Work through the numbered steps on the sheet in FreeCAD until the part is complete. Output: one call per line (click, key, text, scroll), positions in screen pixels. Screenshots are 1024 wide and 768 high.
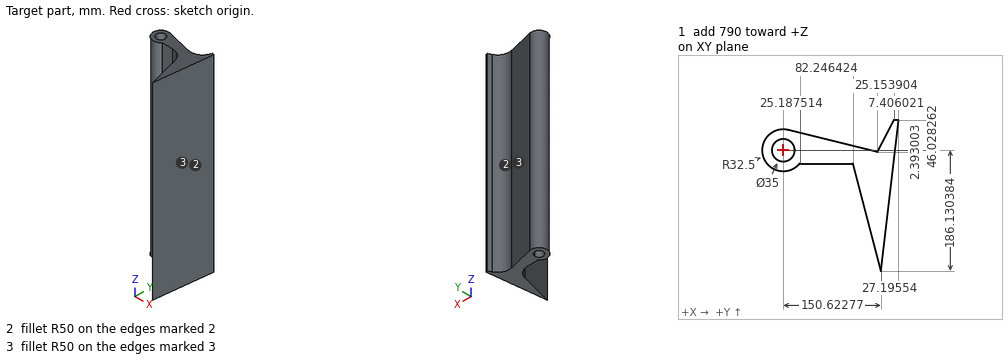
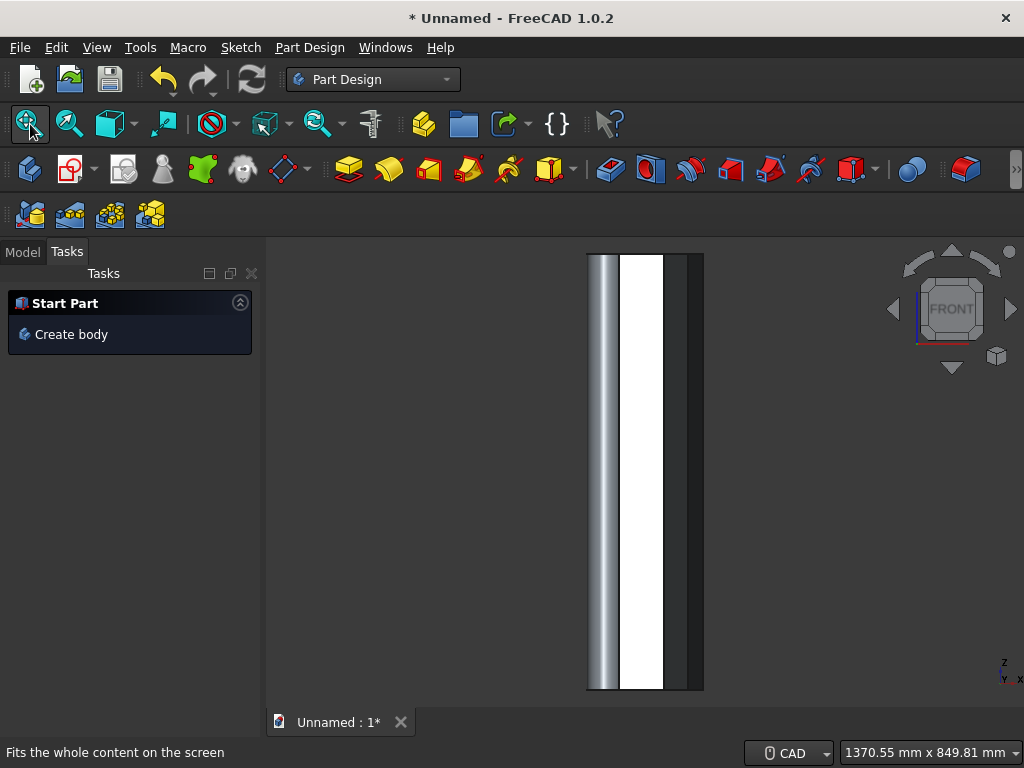
key(3)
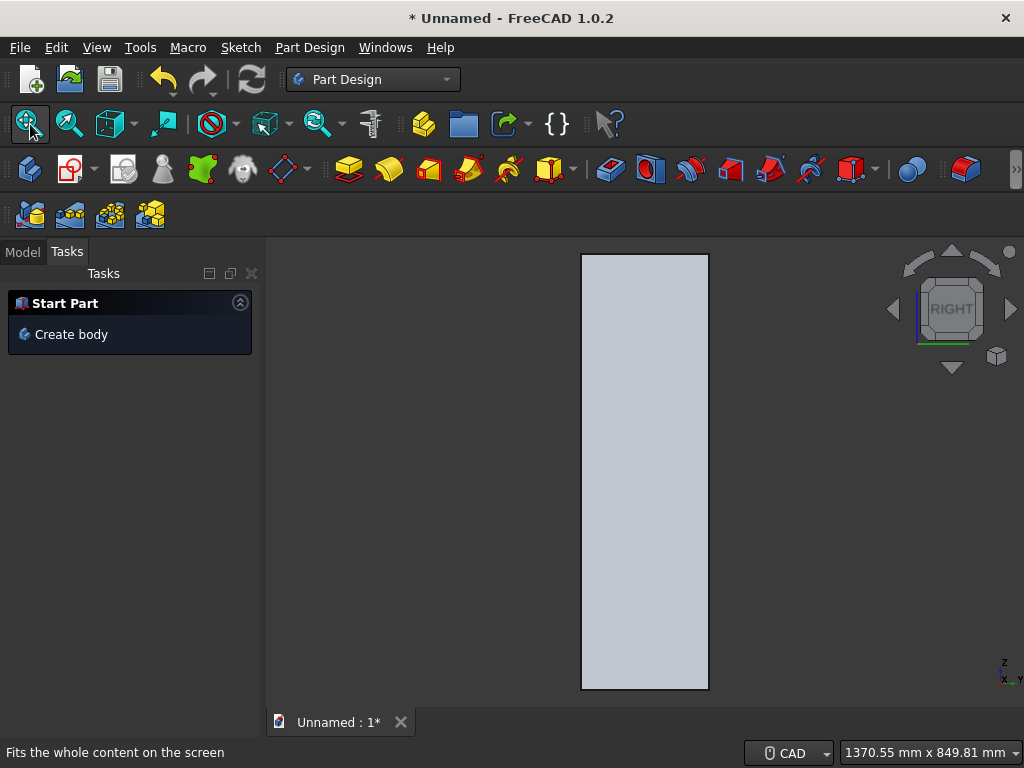
key(5)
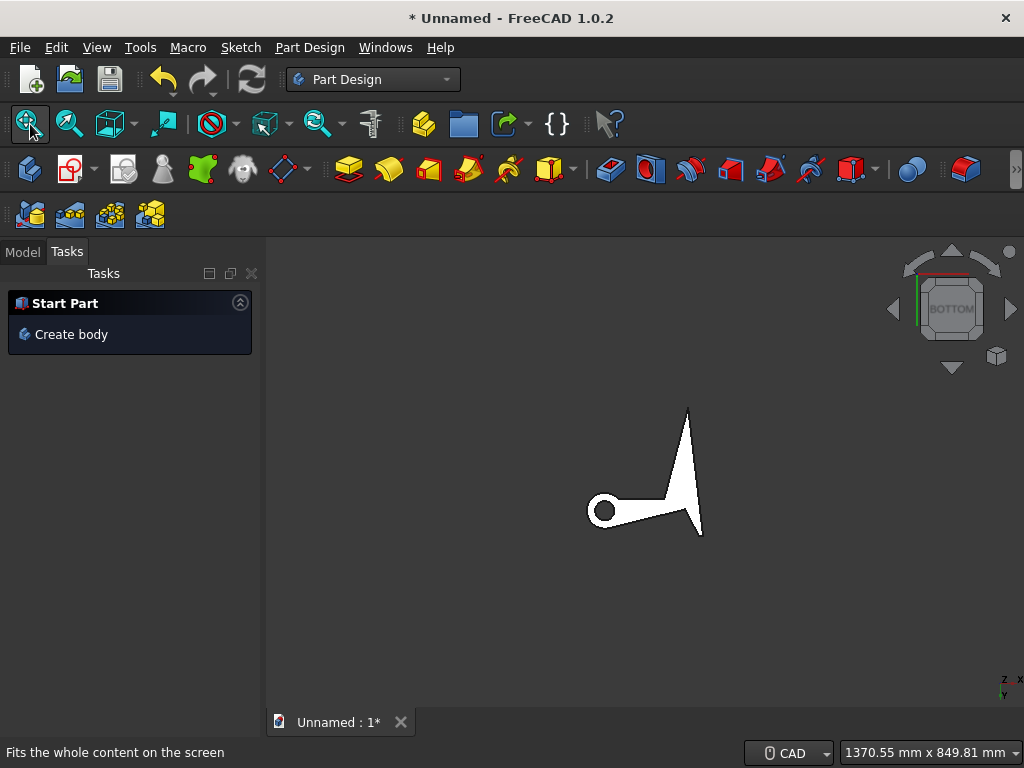
key(v)
key(f)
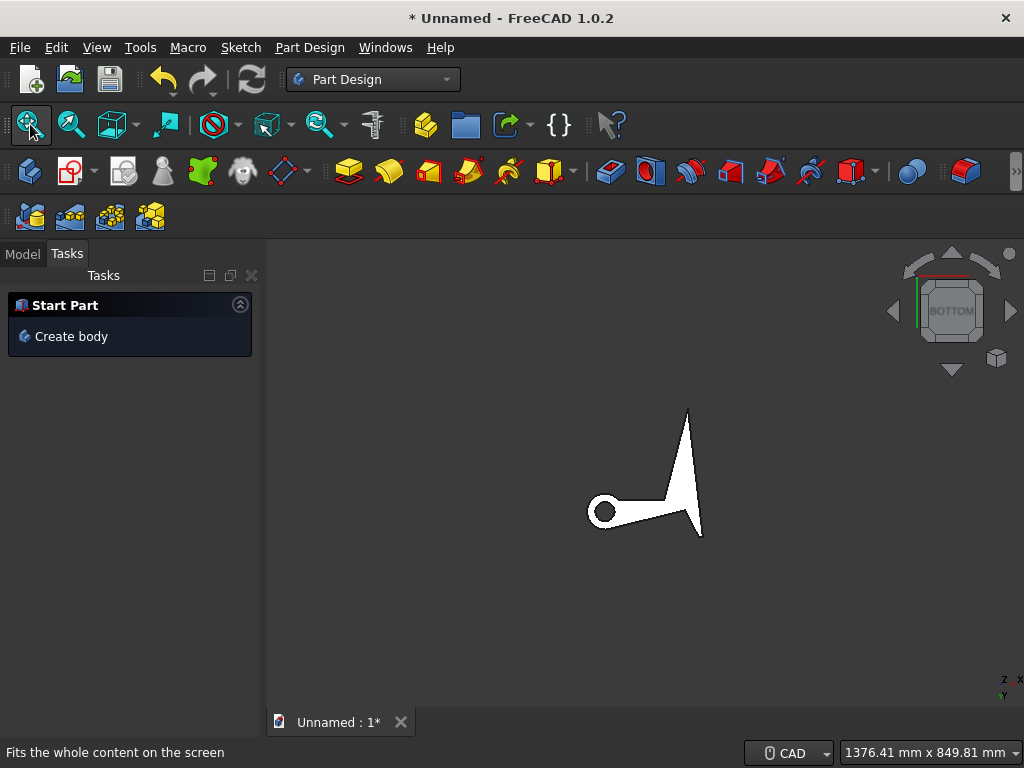
key(4)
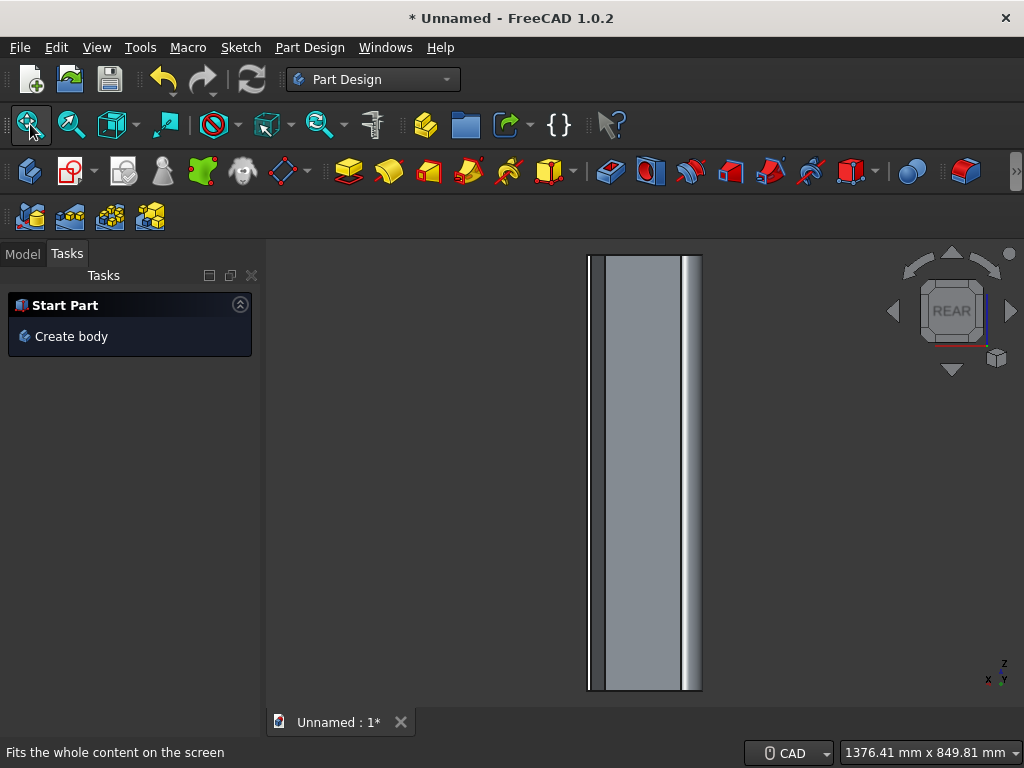
key(6)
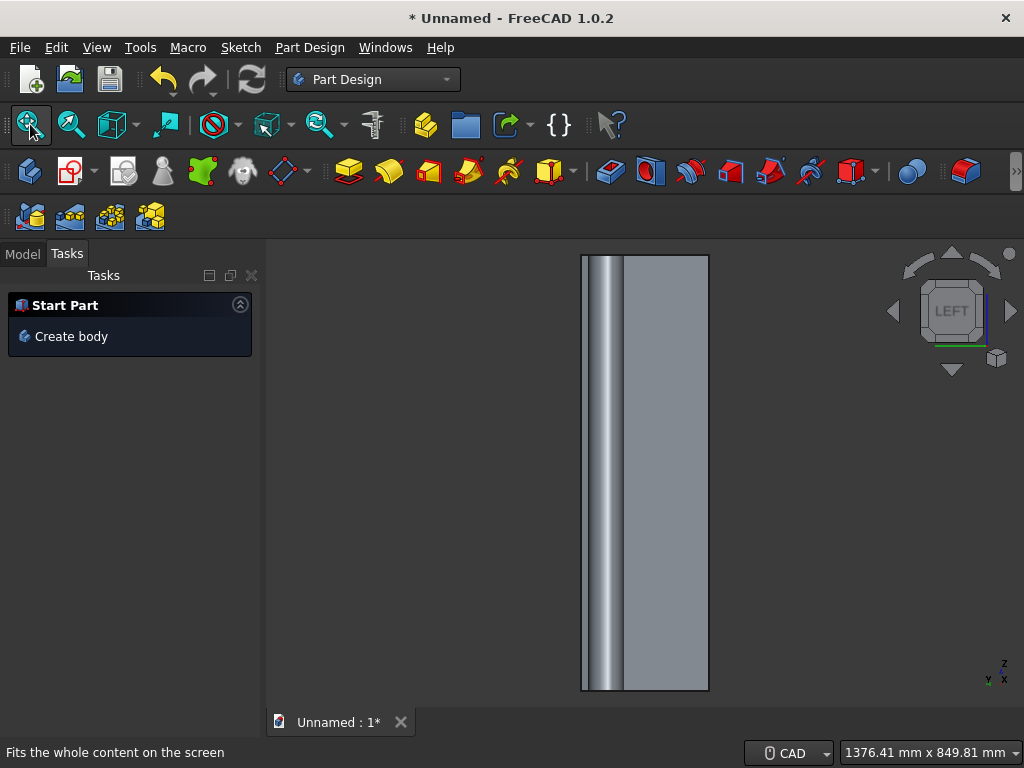
key(v)
key(3)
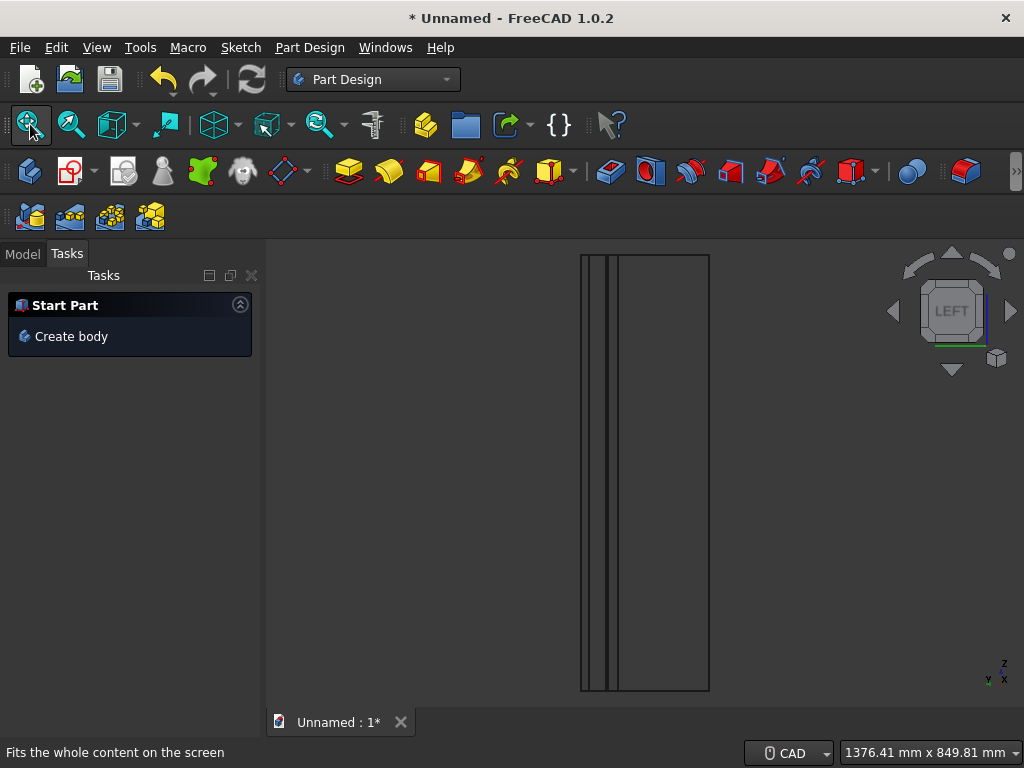
key(0)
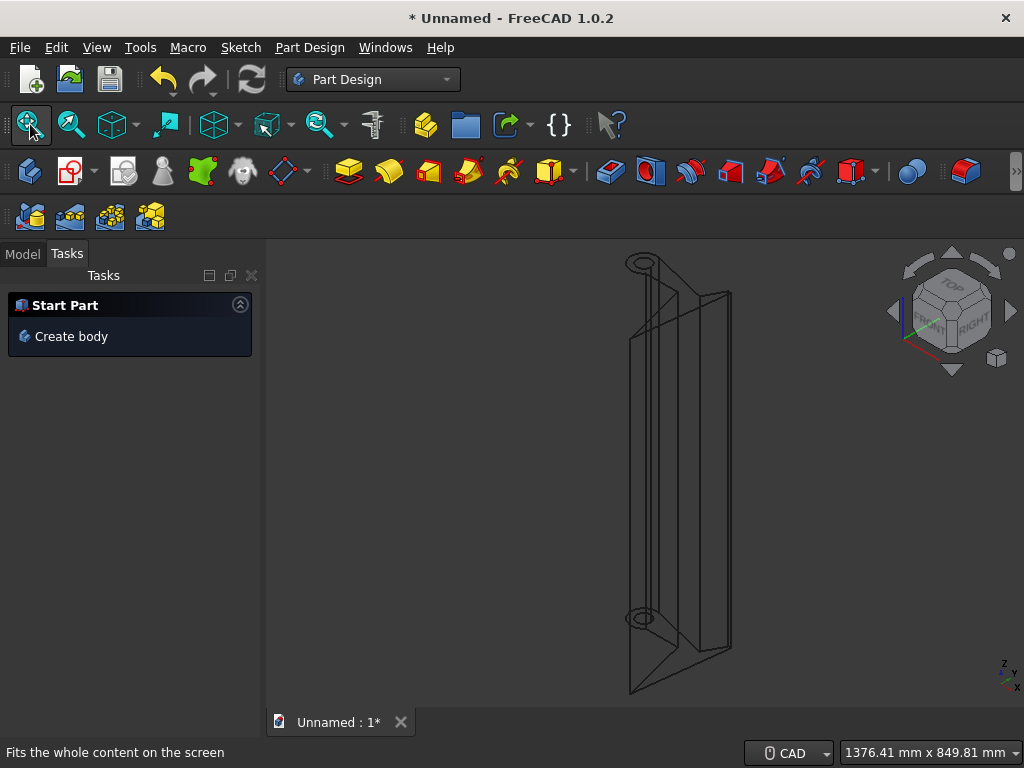
click(700, 473)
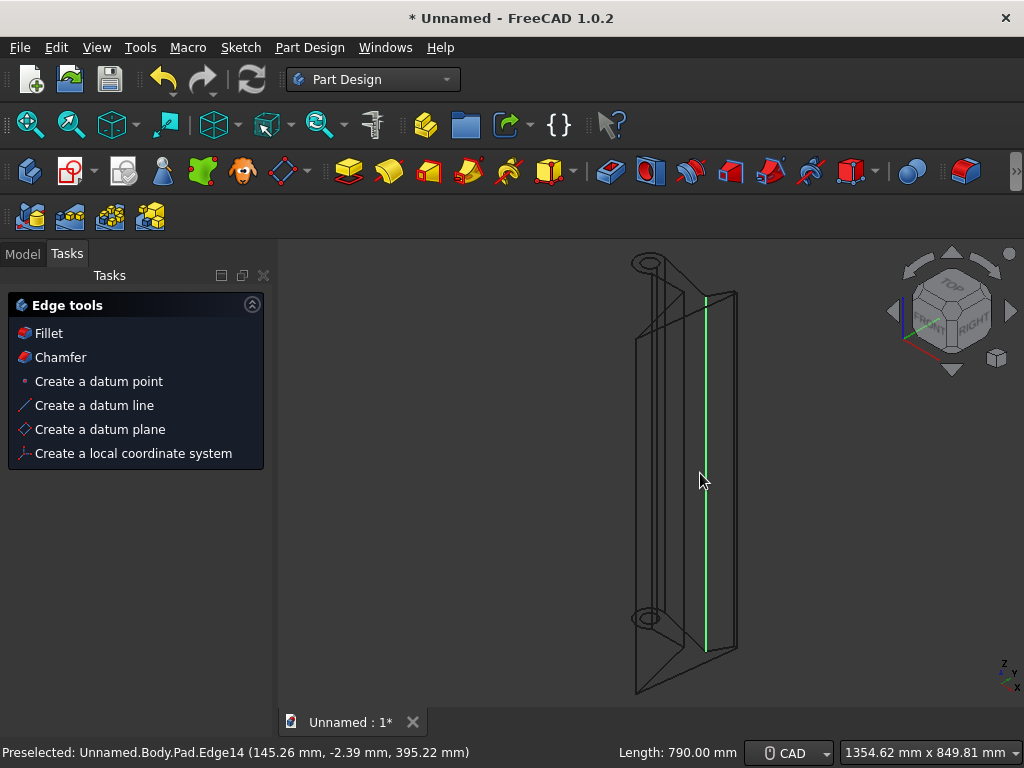
key(v)
key(1)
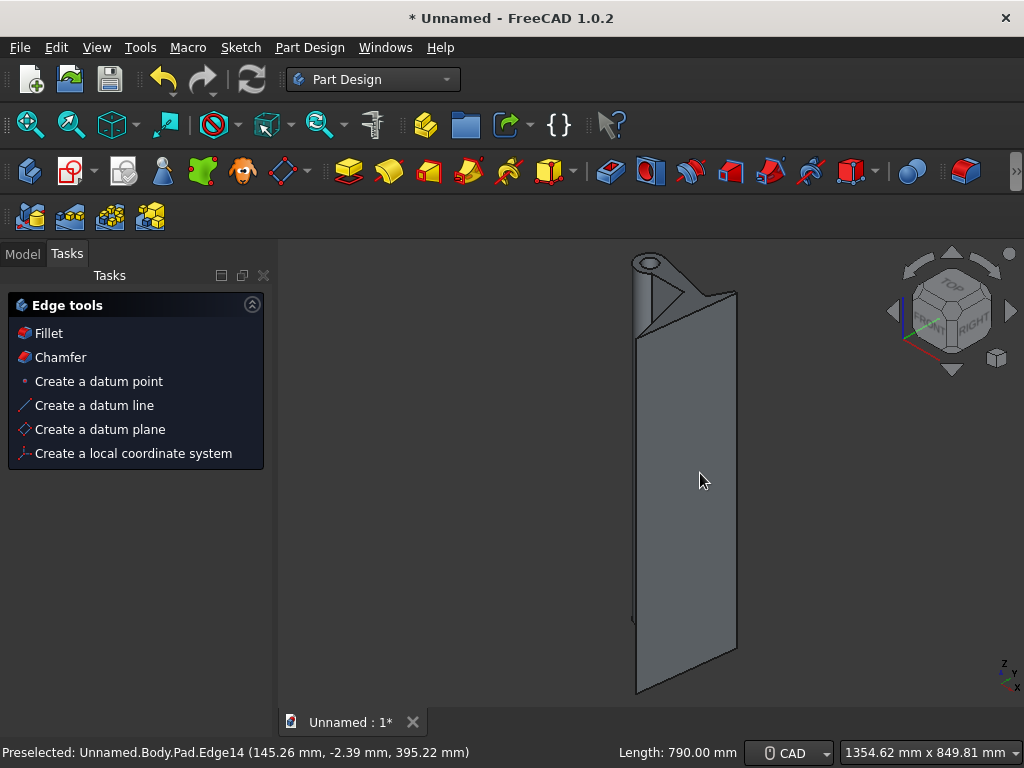
click(966, 172)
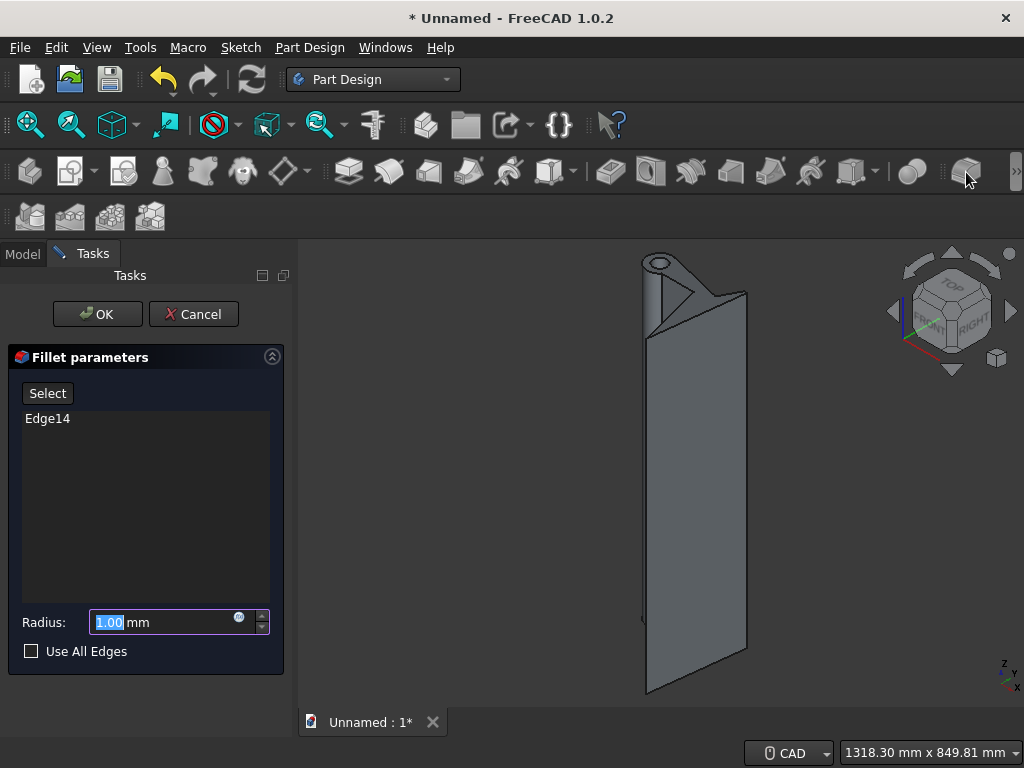
text(50)
key(Tab)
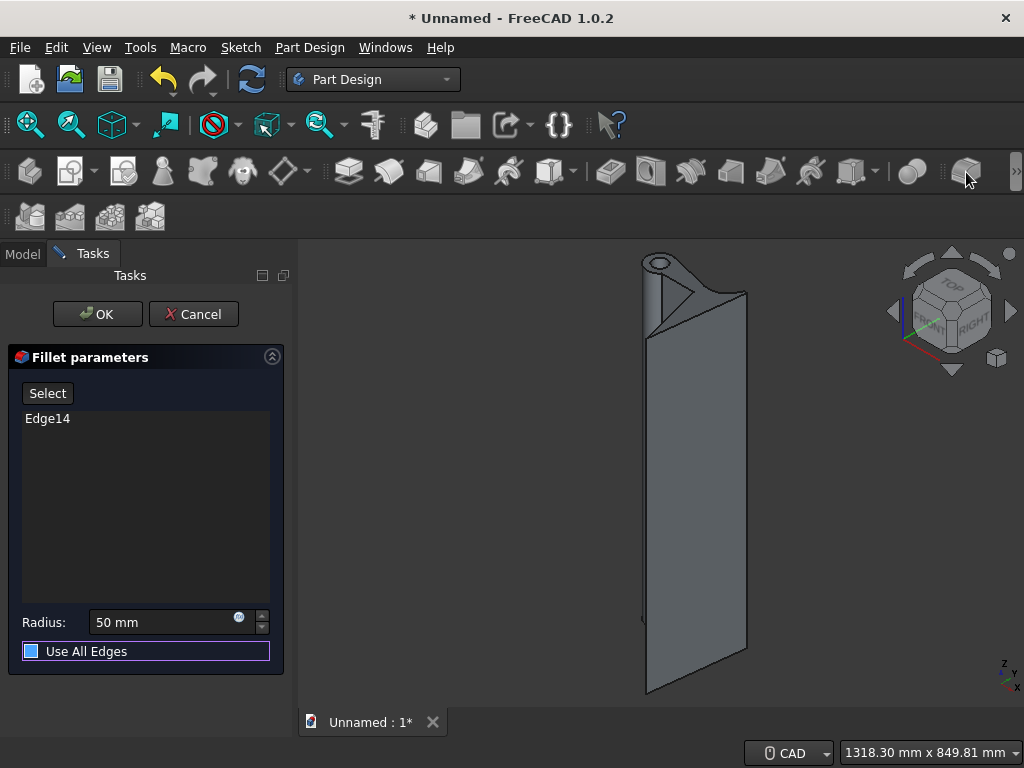
click(98, 314)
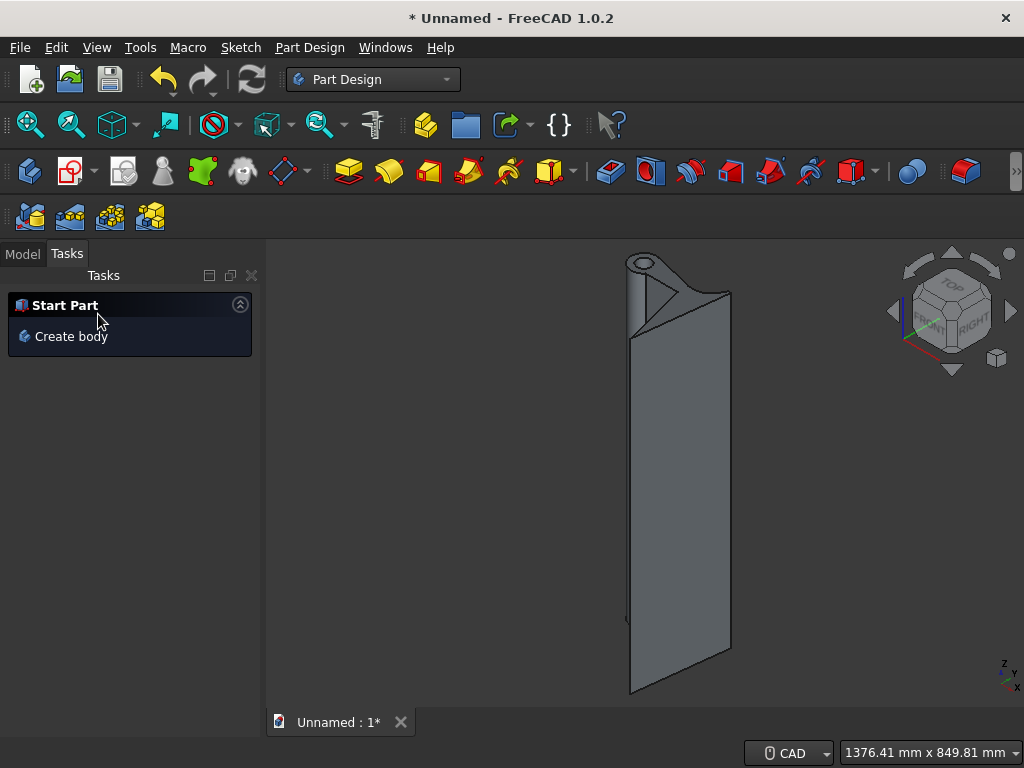
key(2)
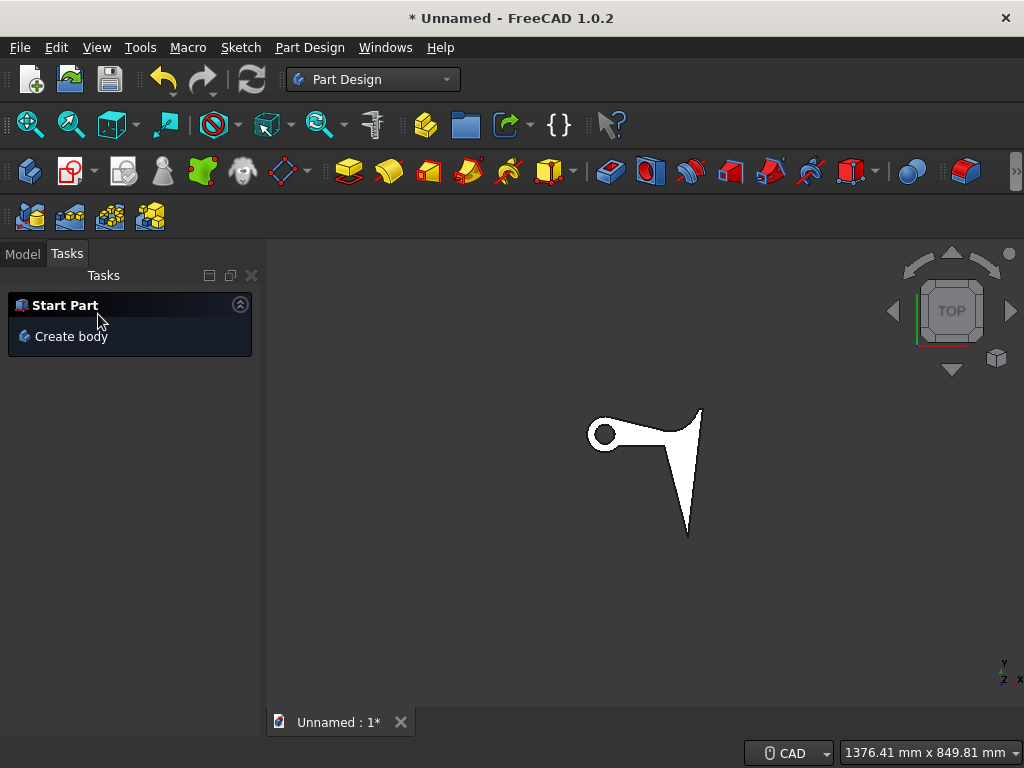
key(v)
key(f)